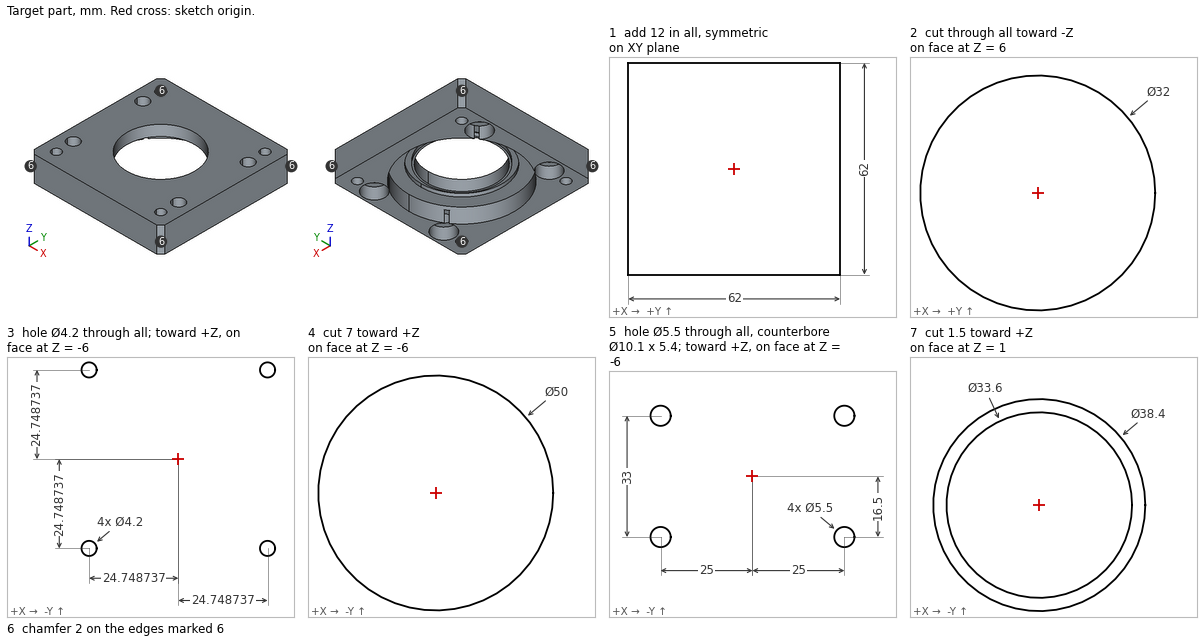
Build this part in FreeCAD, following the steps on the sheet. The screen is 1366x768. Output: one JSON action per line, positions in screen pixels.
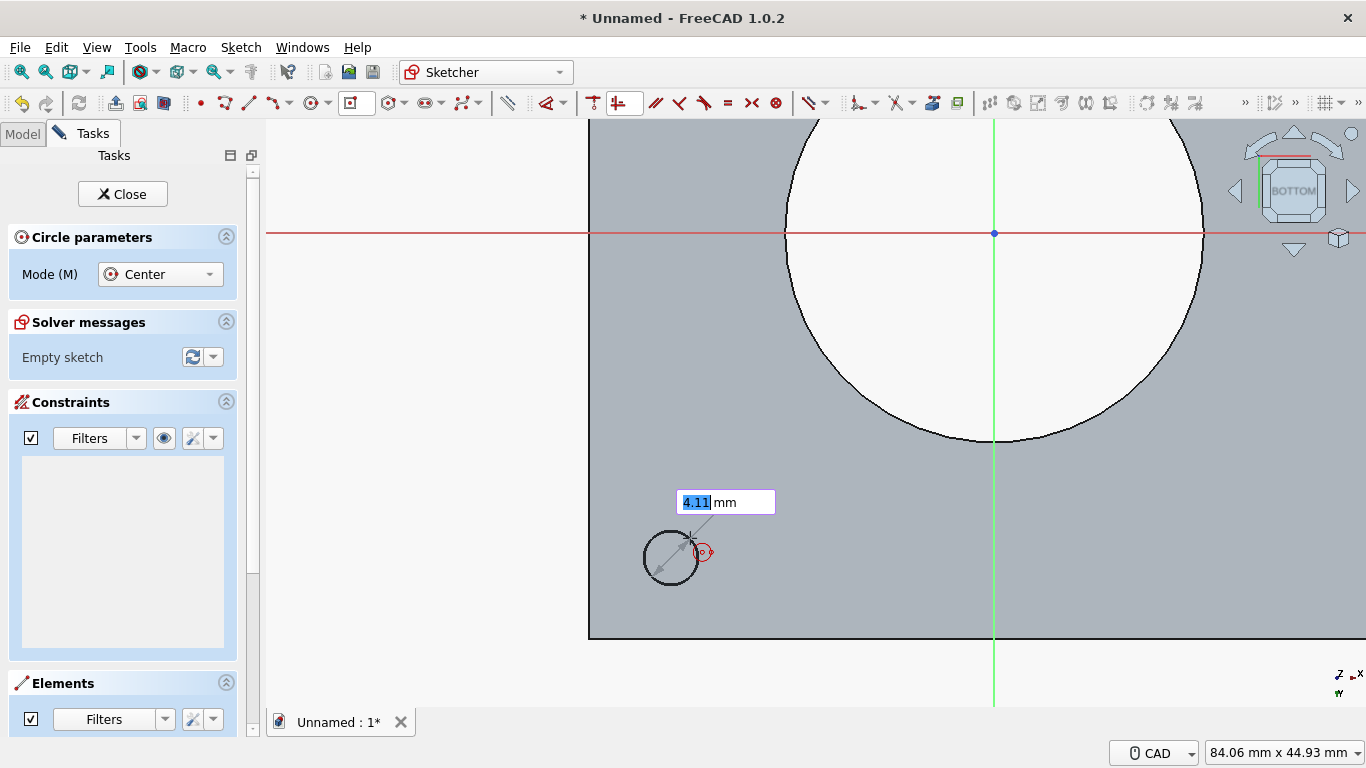
{"action": "type", "text": "4.2"}
{"action": "key", "text": "Return"}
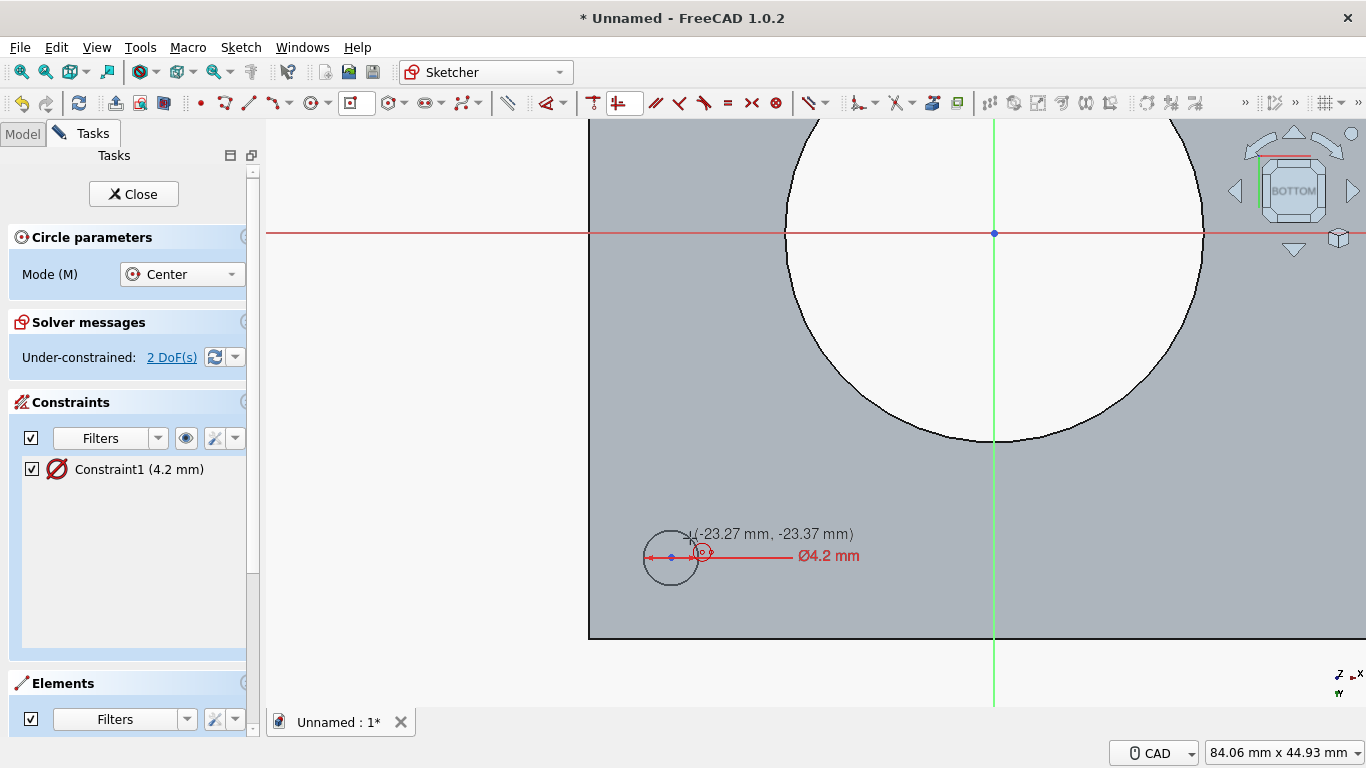
{"action": "scroll", "coordinate": [447, 632], "scroll_direction": "down", "scroll_amount": 3}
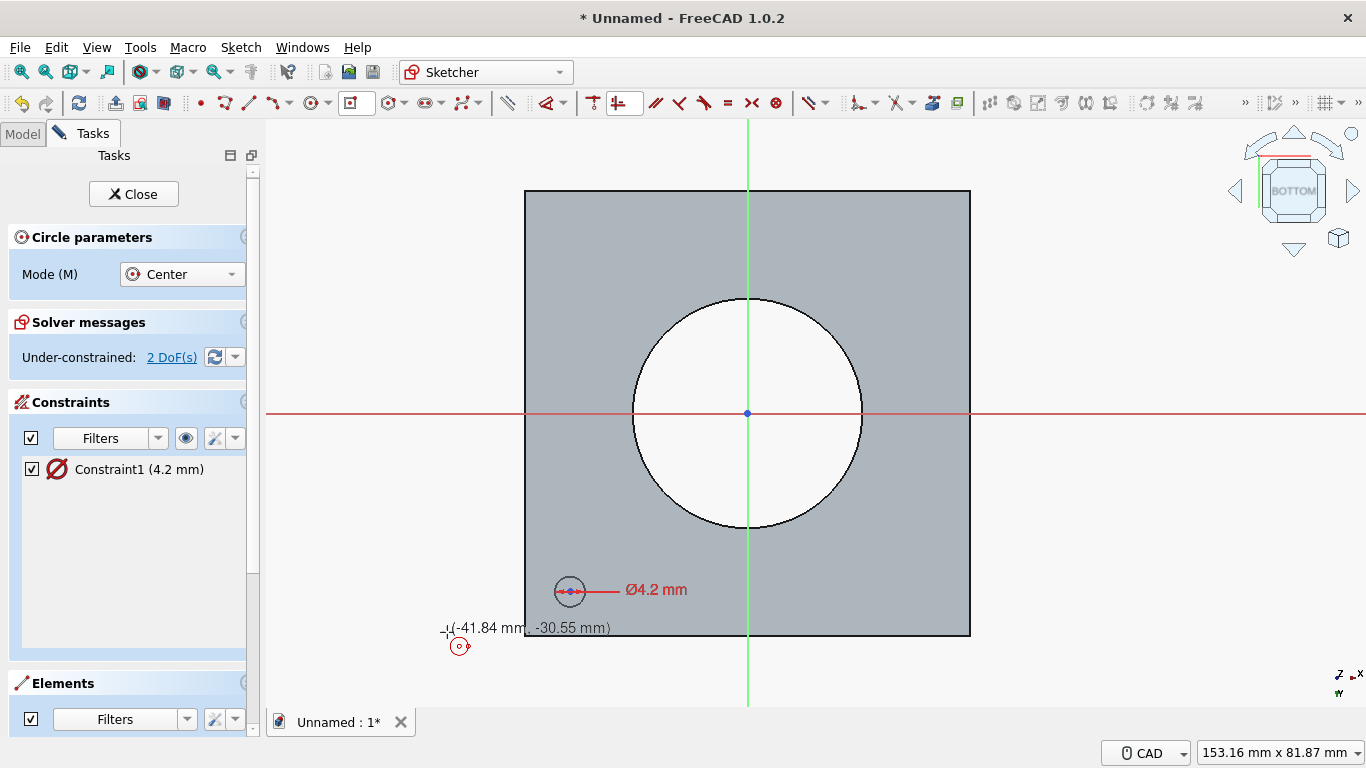
{"action": "scroll", "coordinate": [925, 591], "scroll_direction": "up", "scroll_amount": 3}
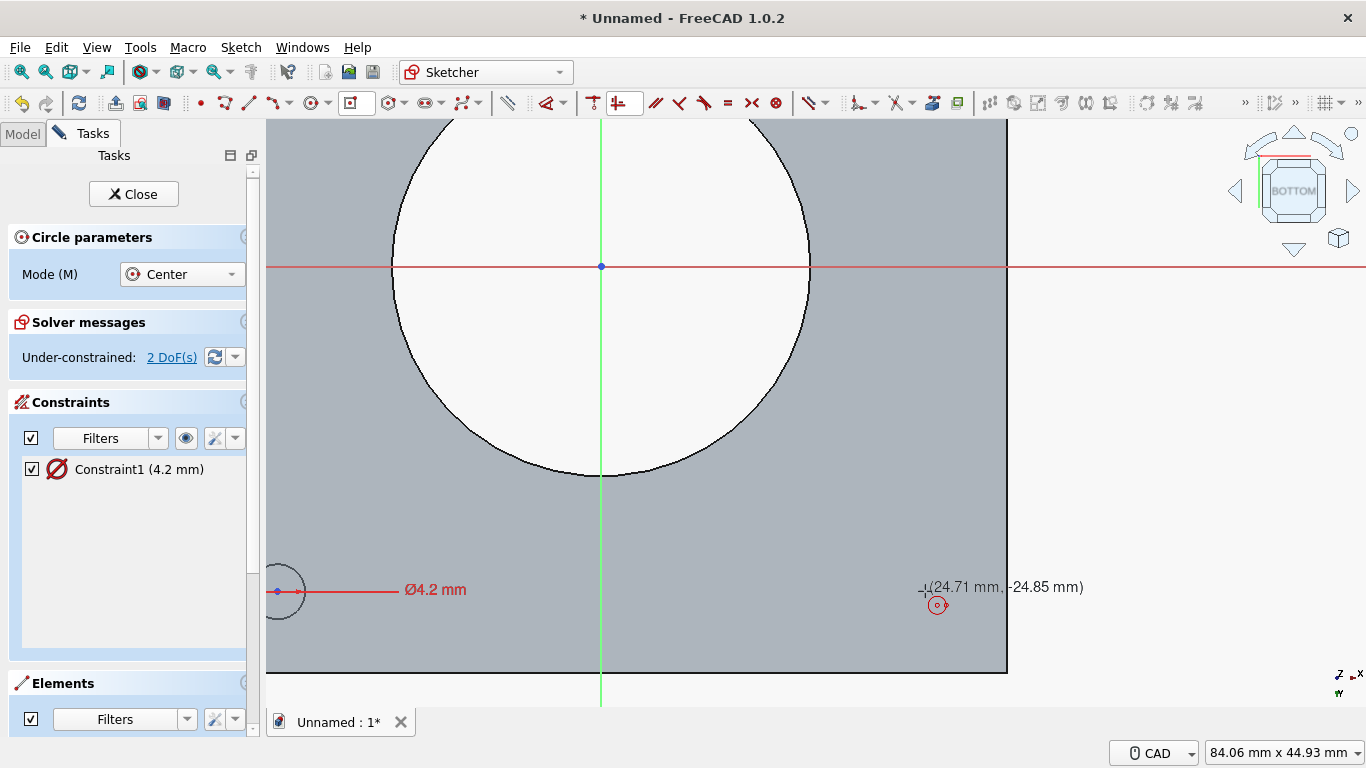
{"action": "left_click", "coordinate": [925, 591]}
{"action": "mouse_move", "coordinate": [944, 571]}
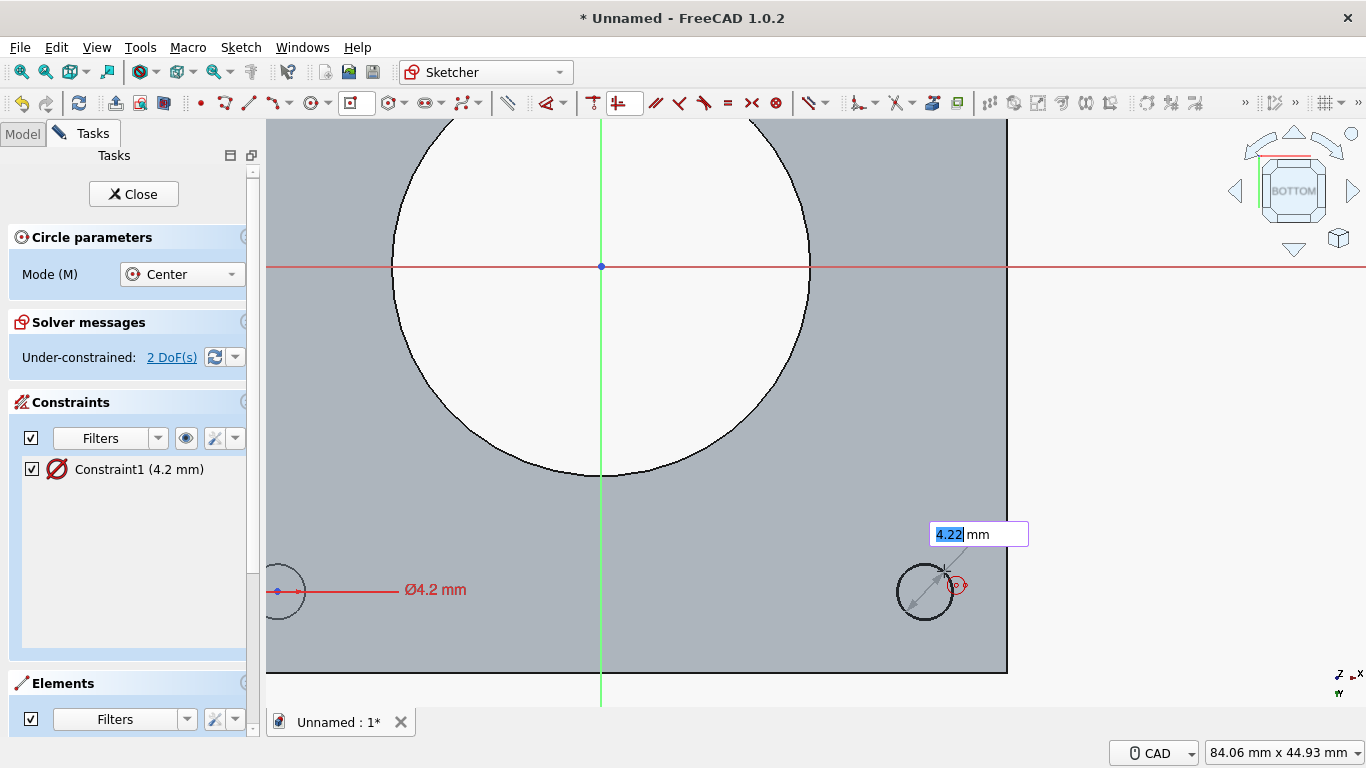
{"action": "type", "text": "4.2"}
{"action": "key", "text": "Return"}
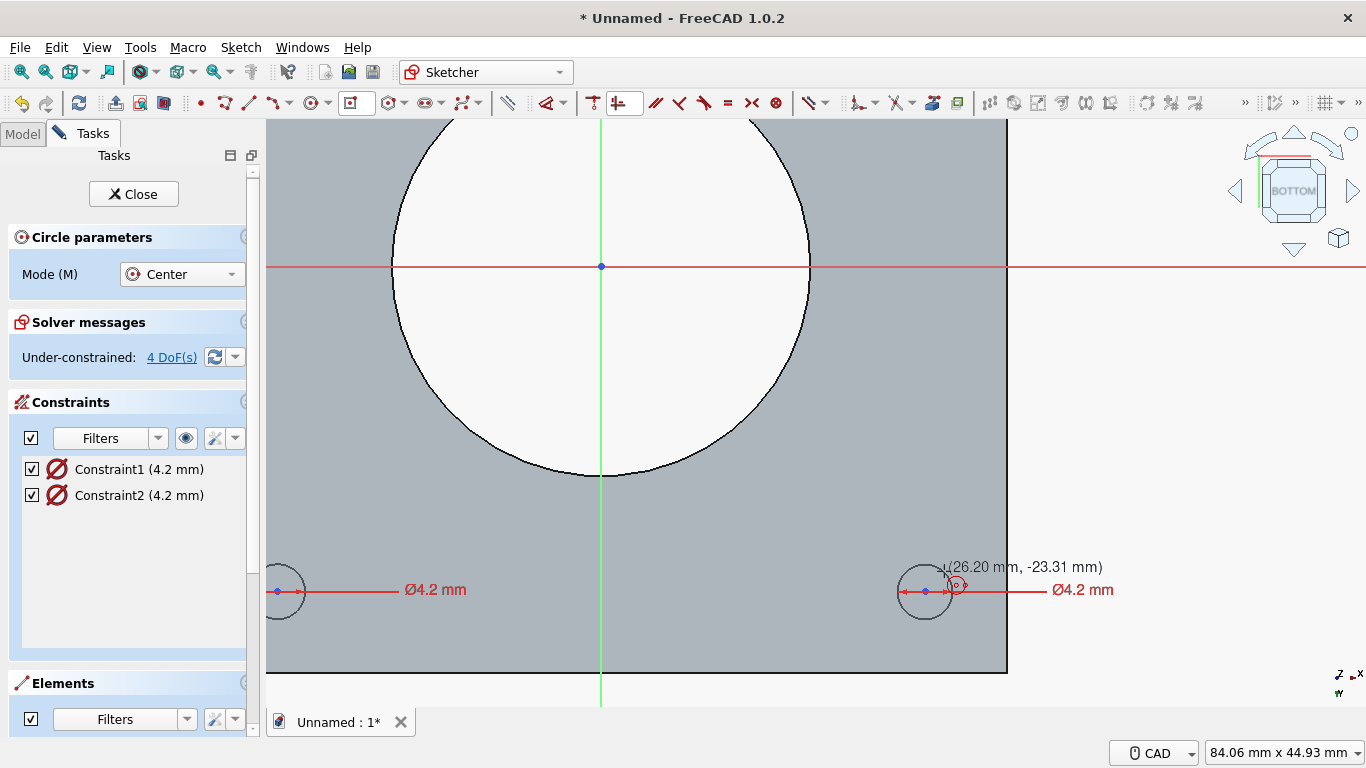
{"action": "scroll", "coordinate": [926, 591], "scroll_direction": "down", "scroll_amount": 3}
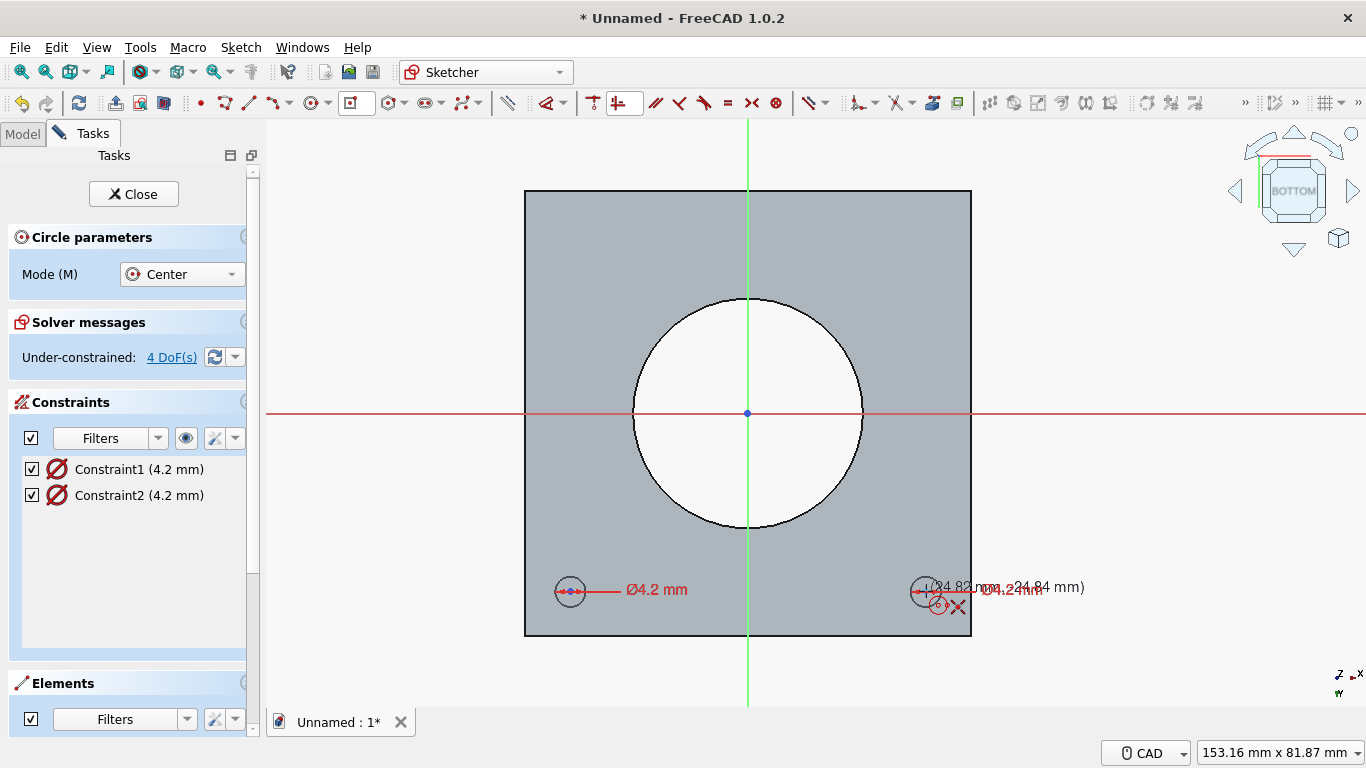
{"action": "scroll", "coordinate": [570, 236], "scroll_direction": "up", "scroll_amount": 3}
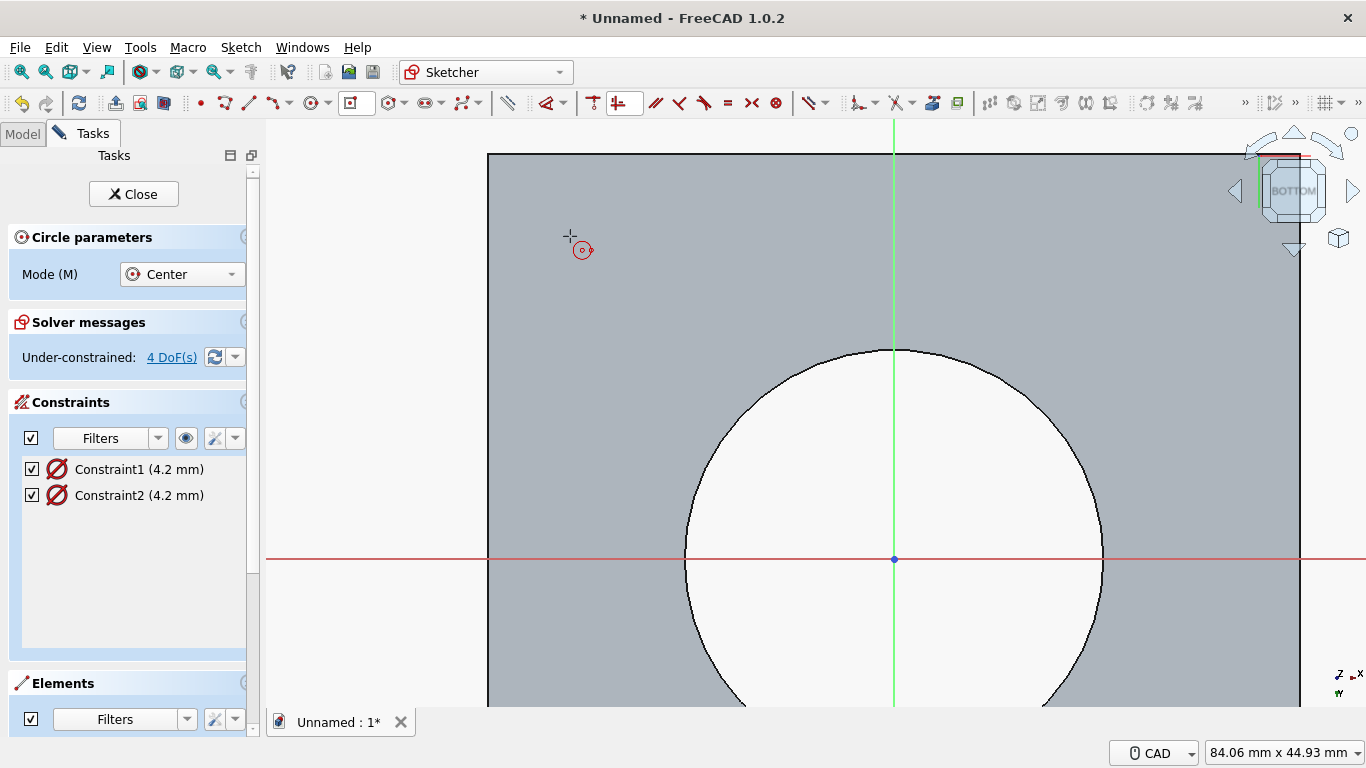
{"action": "left_click", "coordinate": [570, 235]}
{"action": "mouse_move", "coordinate": [590, 216]}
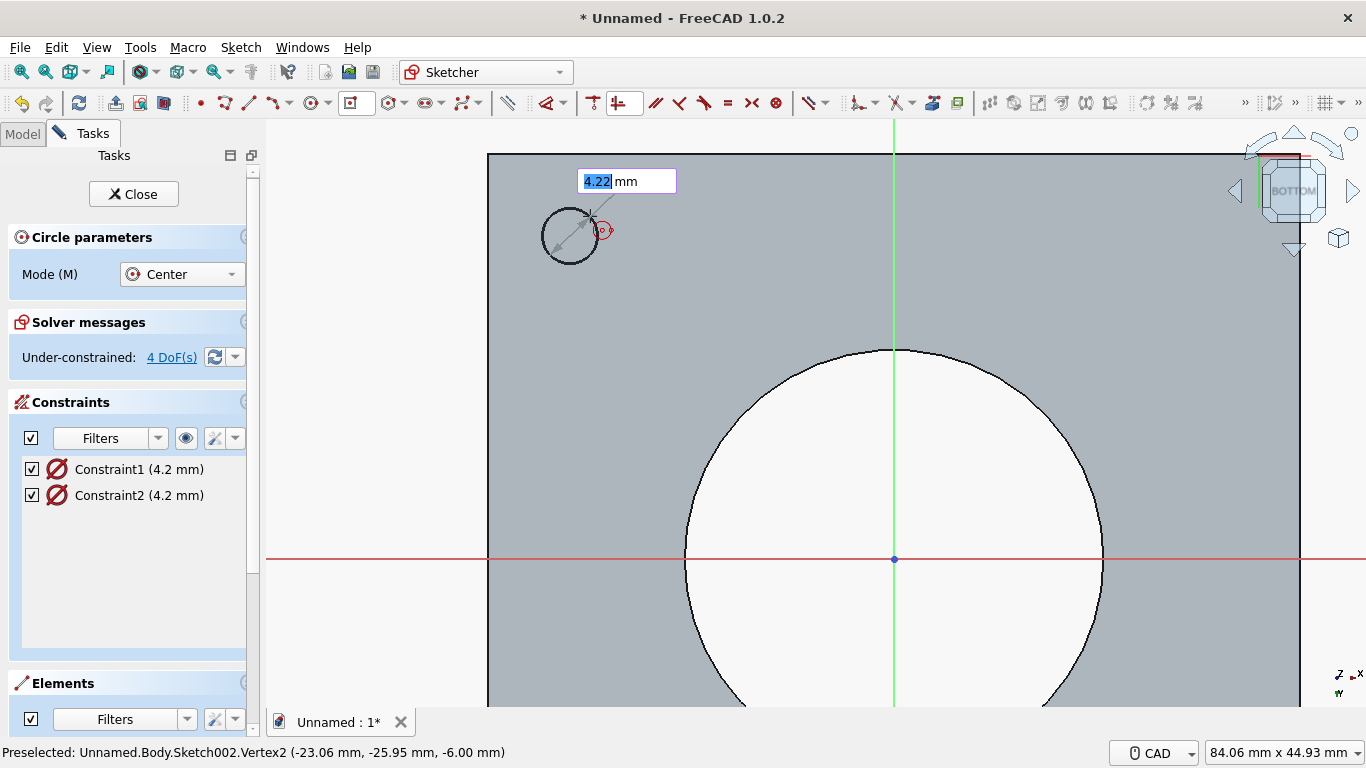
{"action": "type", "text": "4.2"}
{"action": "key", "text": "Return"}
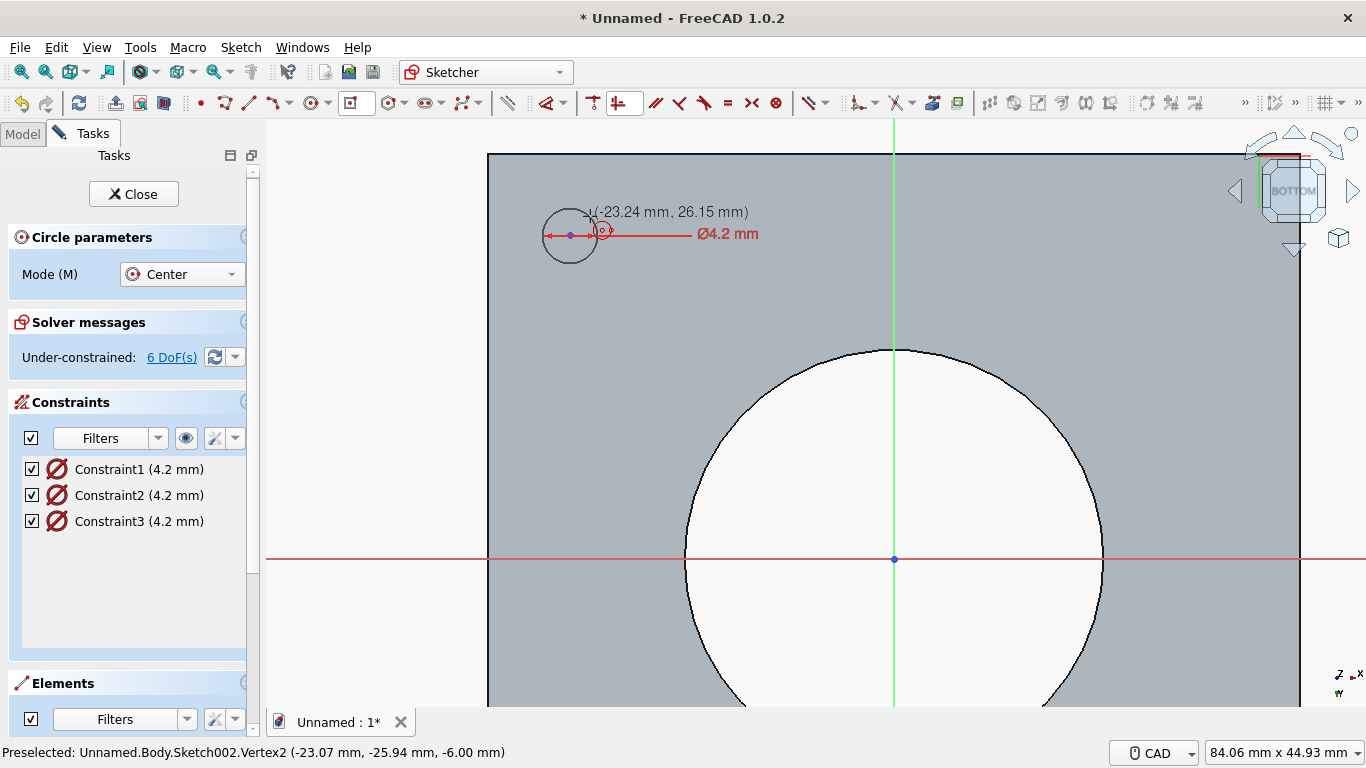
{"action": "scroll", "coordinate": [569, 235], "scroll_direction": "down", "scroll_amount": 3}